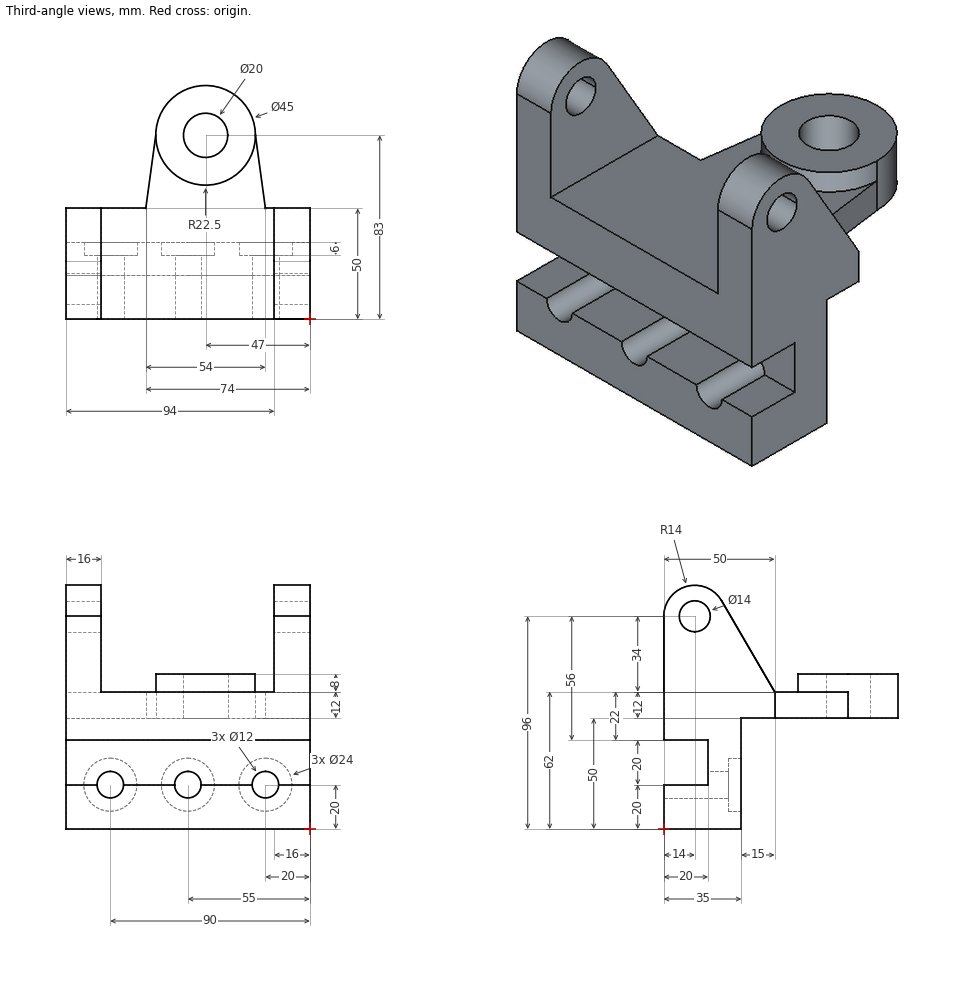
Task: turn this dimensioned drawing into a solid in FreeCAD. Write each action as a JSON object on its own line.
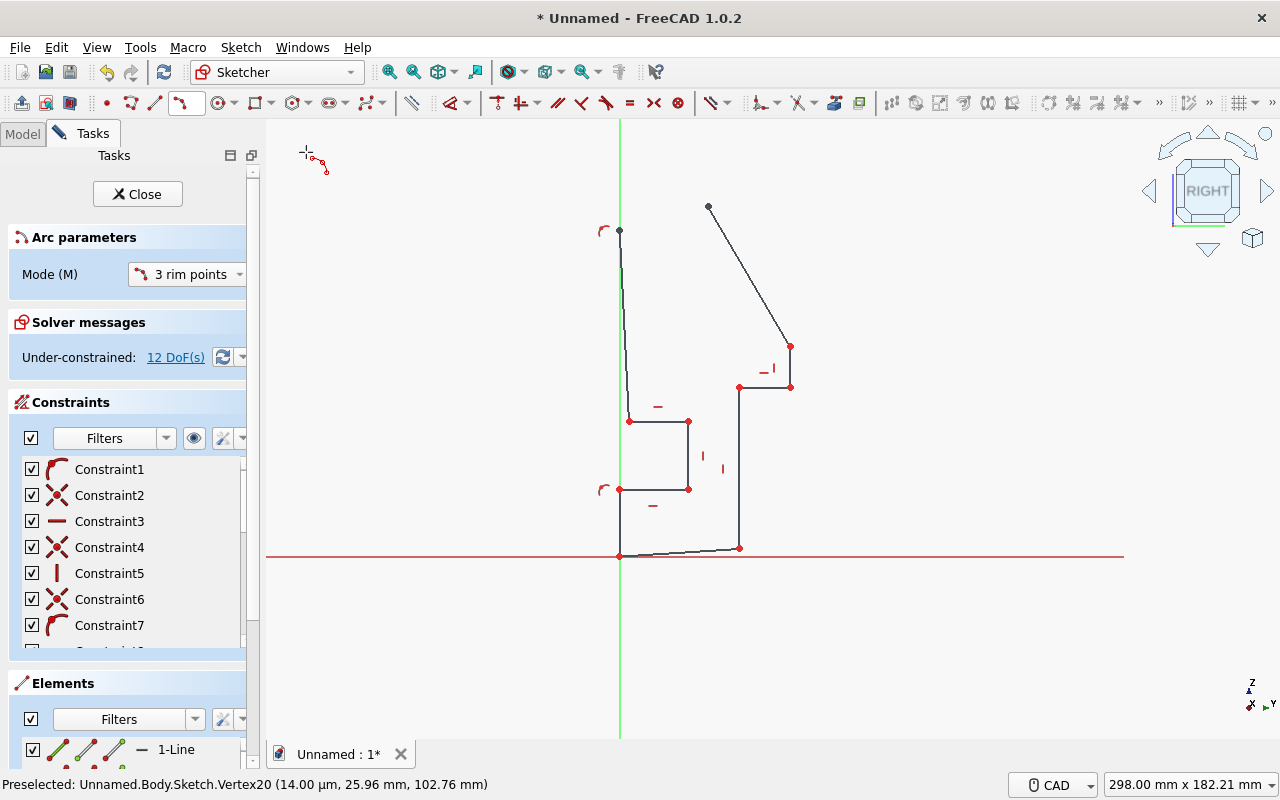
{"action": "left_click", "coordinate": [708, 207]}
{"action": "left_click", "coordinate": [620, 231]}
{"action": "left_click", "coordinate": [655, 184]}
{"action": "key", "text": "Escape"}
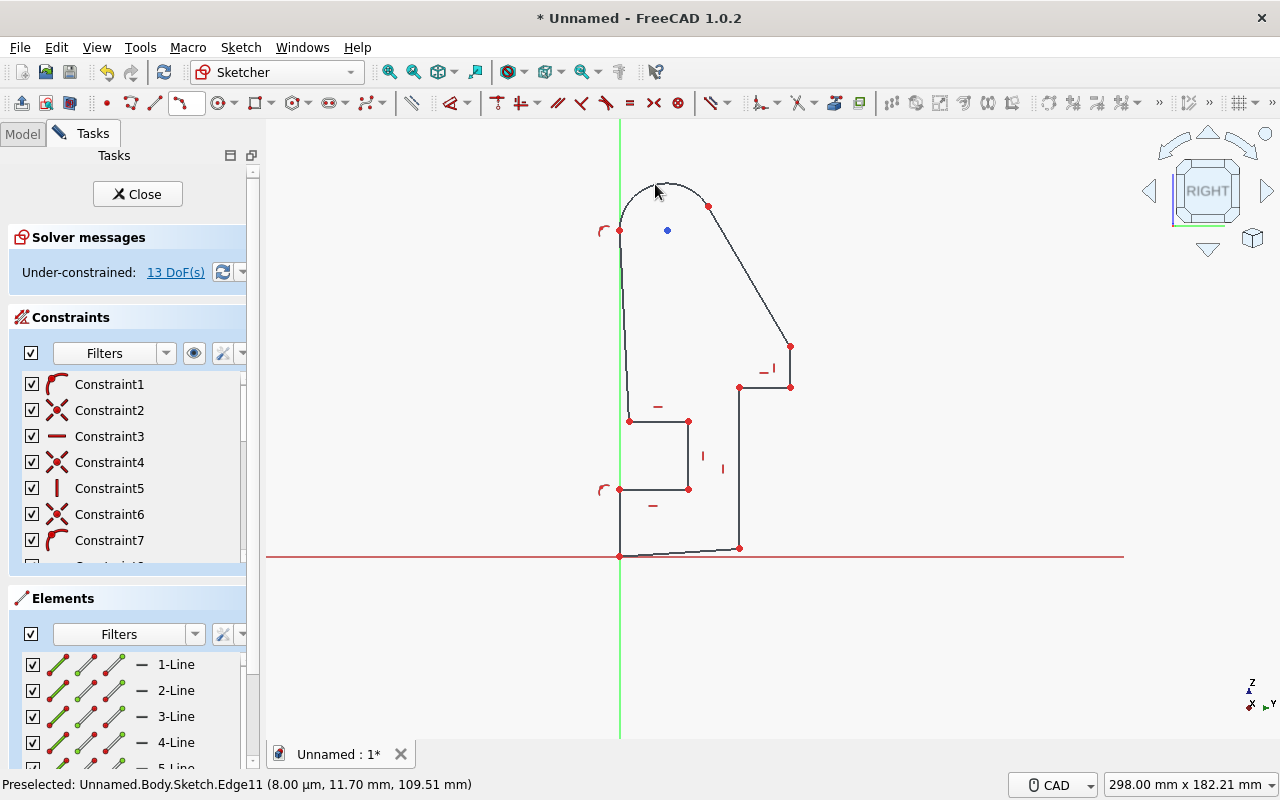
{"action": "left_click", "coordinate": [622, 288]}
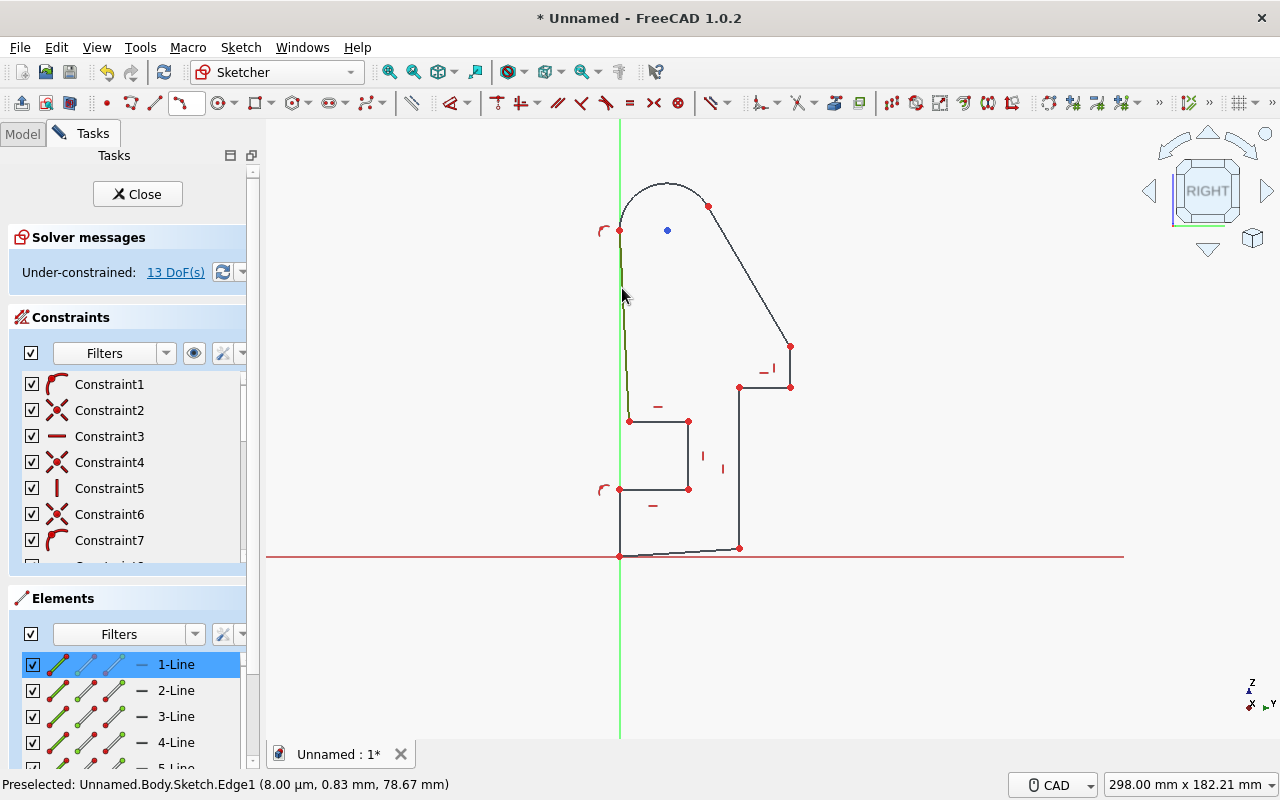
{"action": "left_click", "coordinate": [679, 185]}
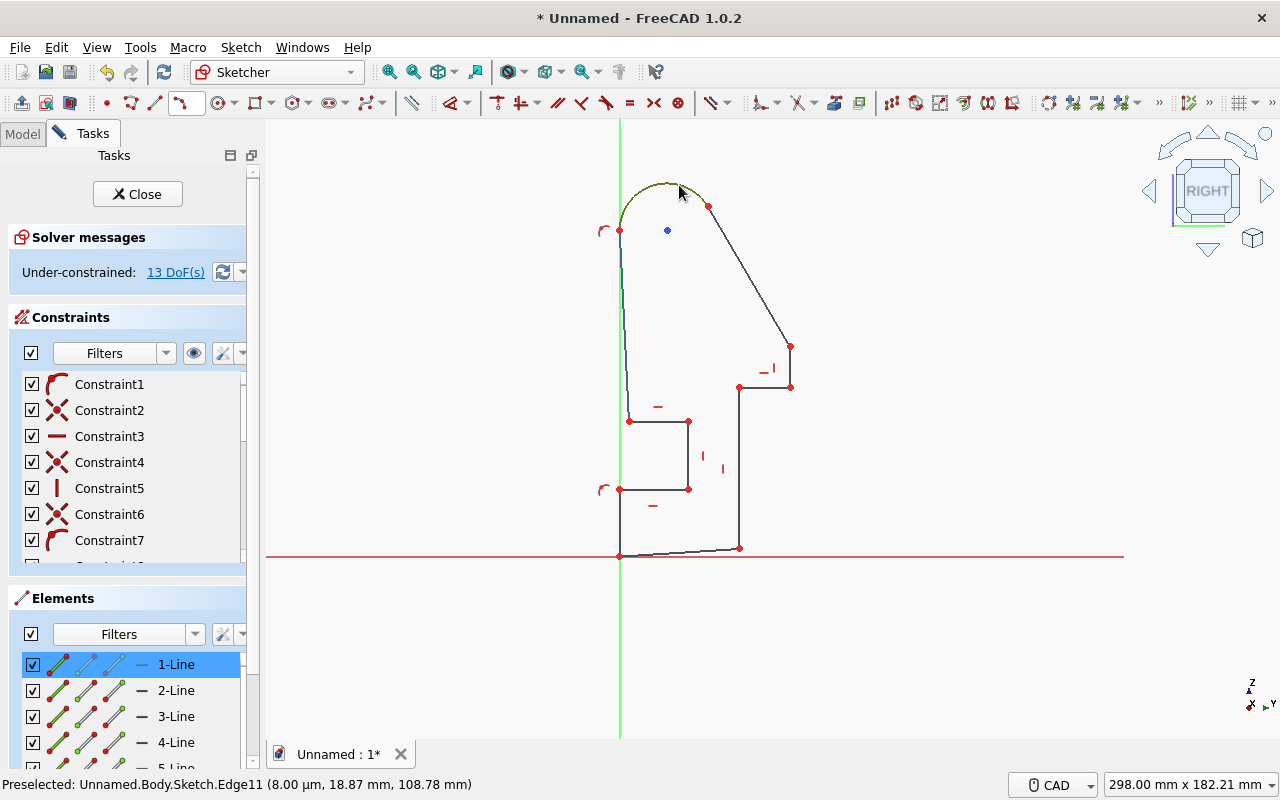
{"action": "left_click", "coordinate": [606, 104]}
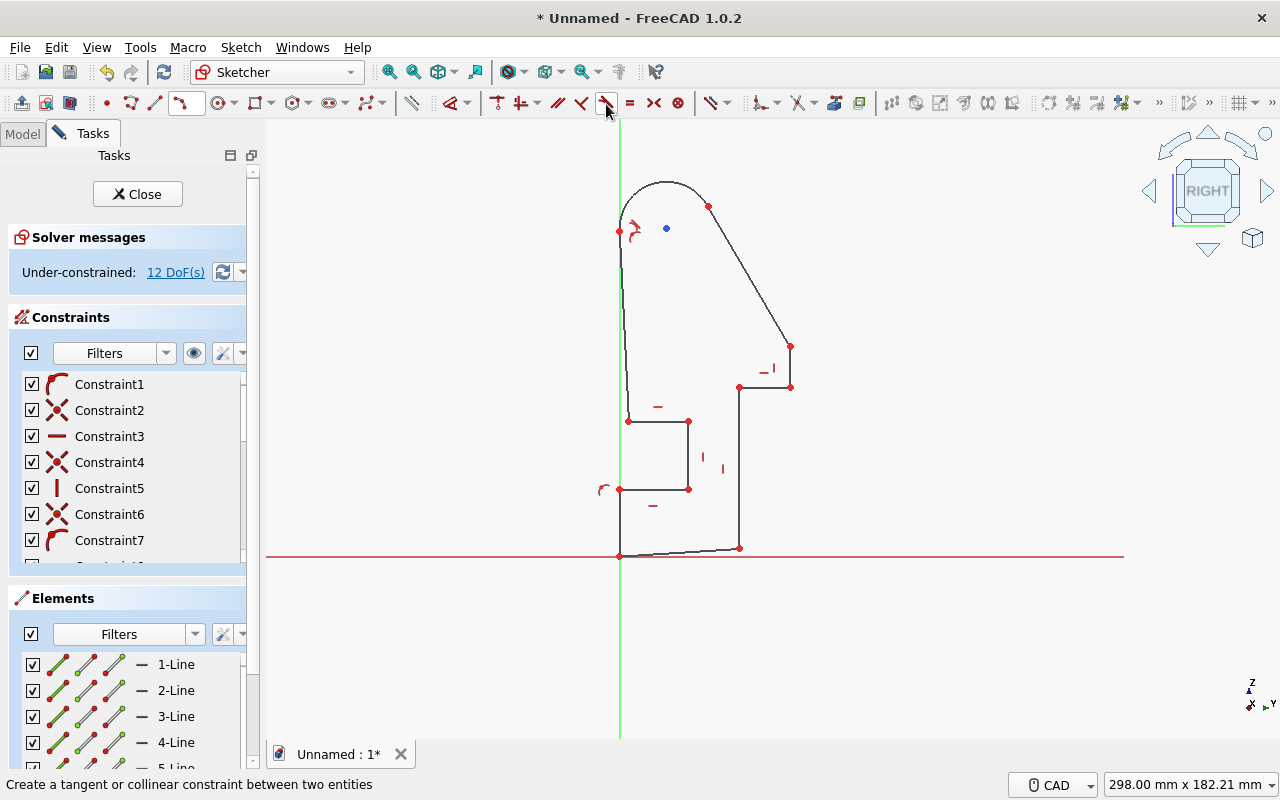
{"action": "left_click", "coordinate": [765, 305]}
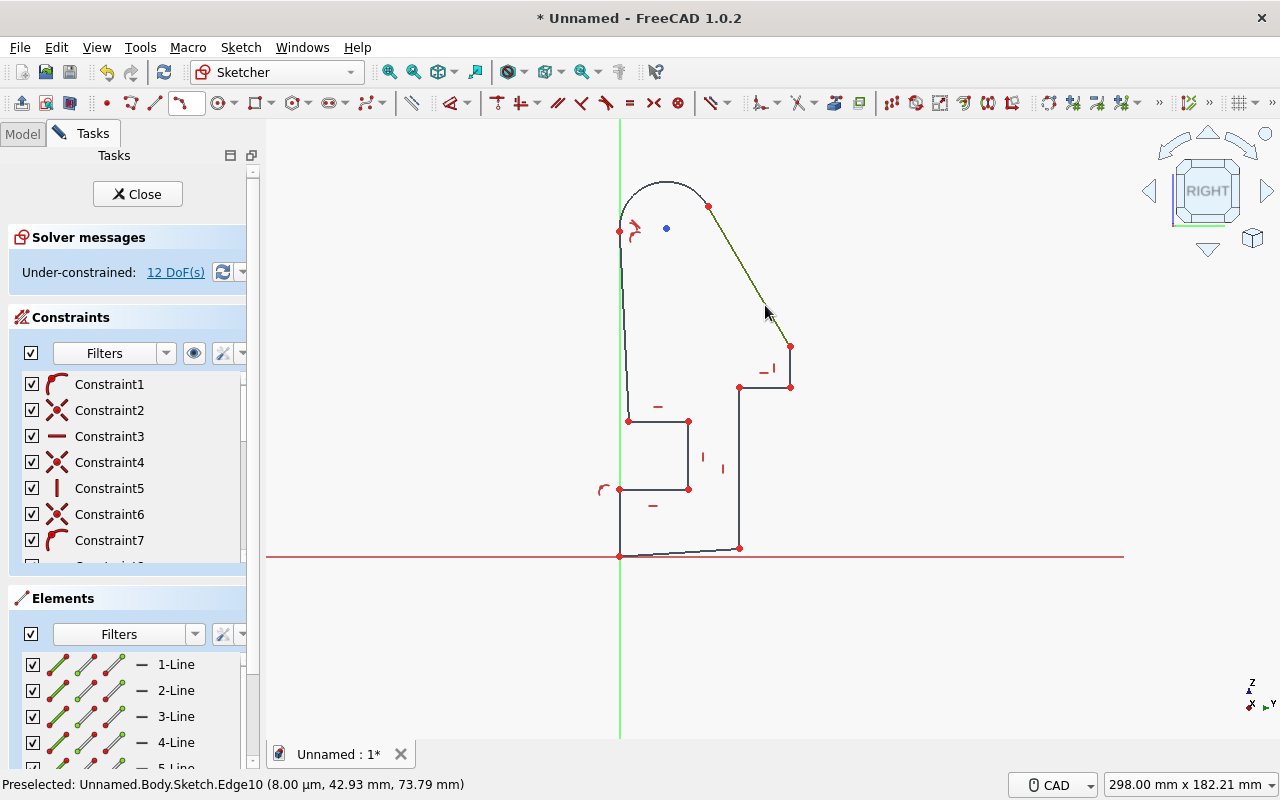
{"action": "left_click", "coordinate": [679, 184]}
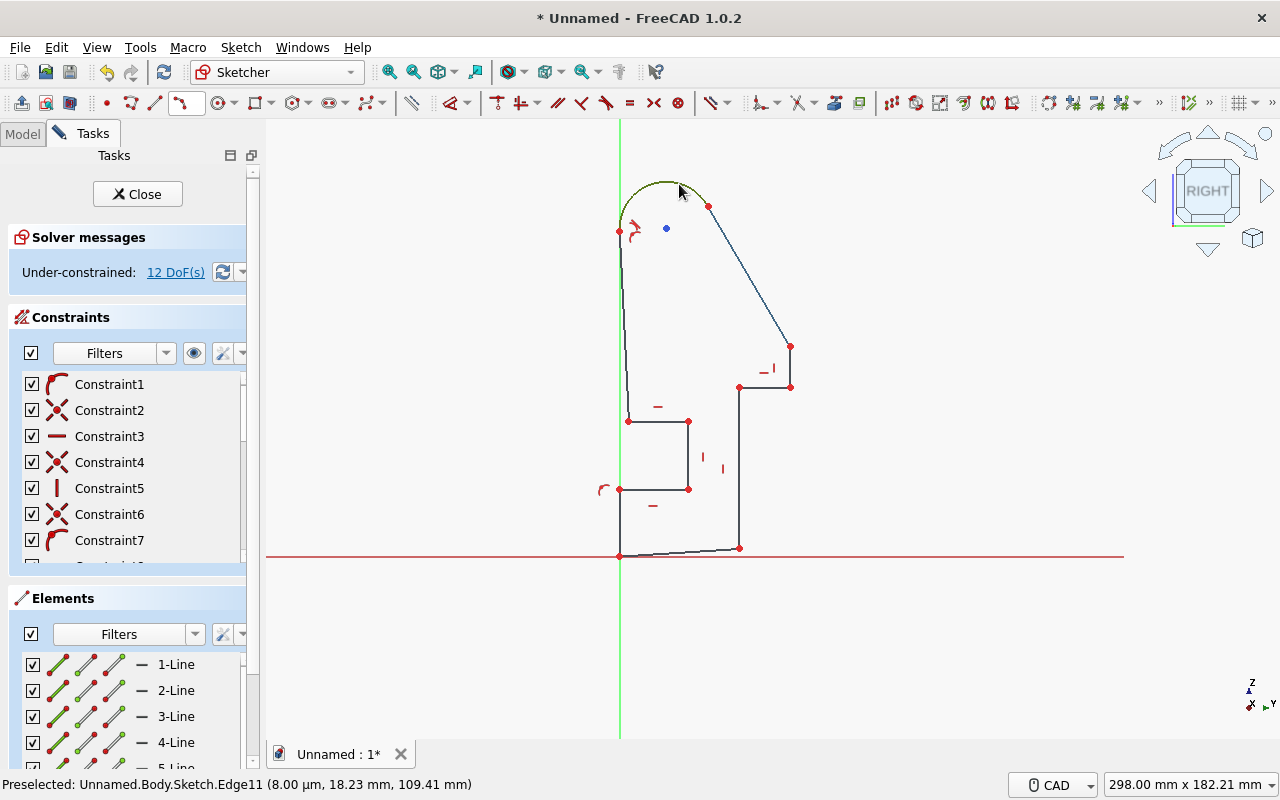
{"action": "left_click", "coordinate": [606, 104]}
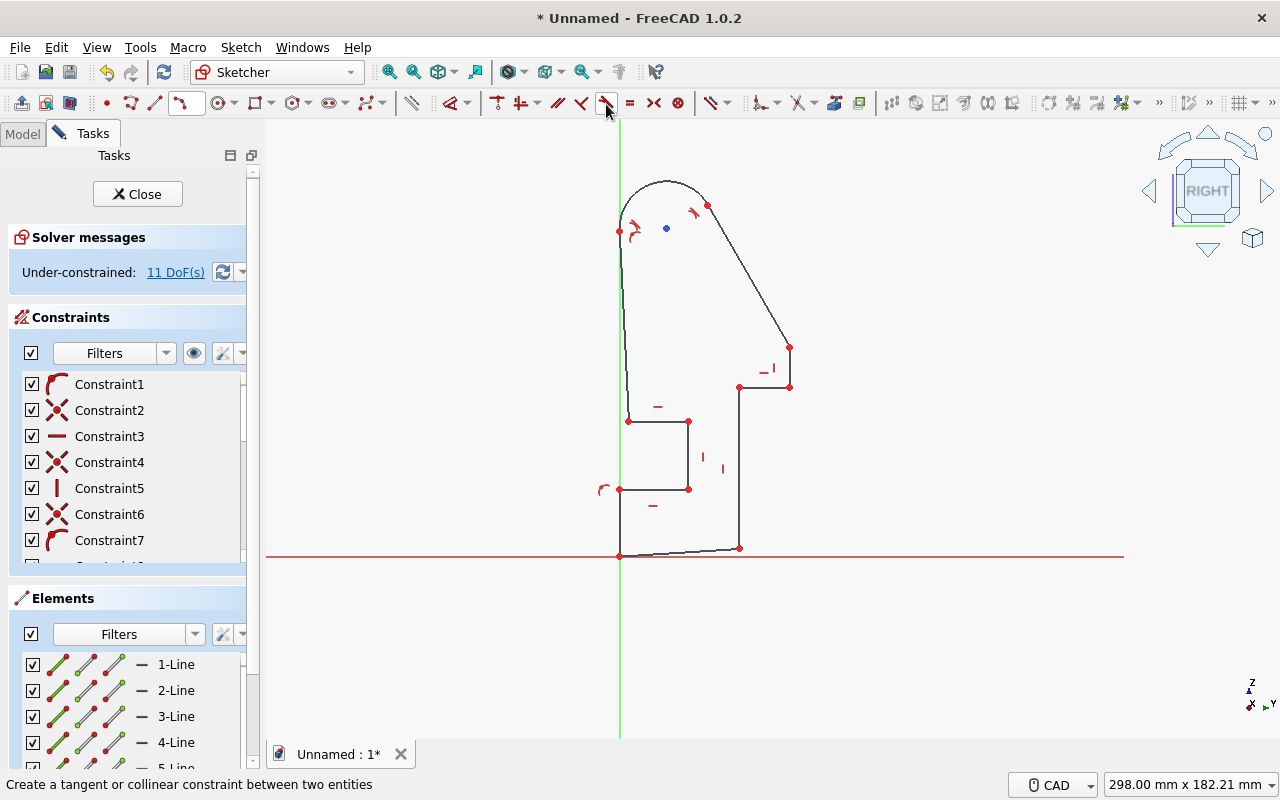
{"action": "left_click", "coordinate": [622, 288]}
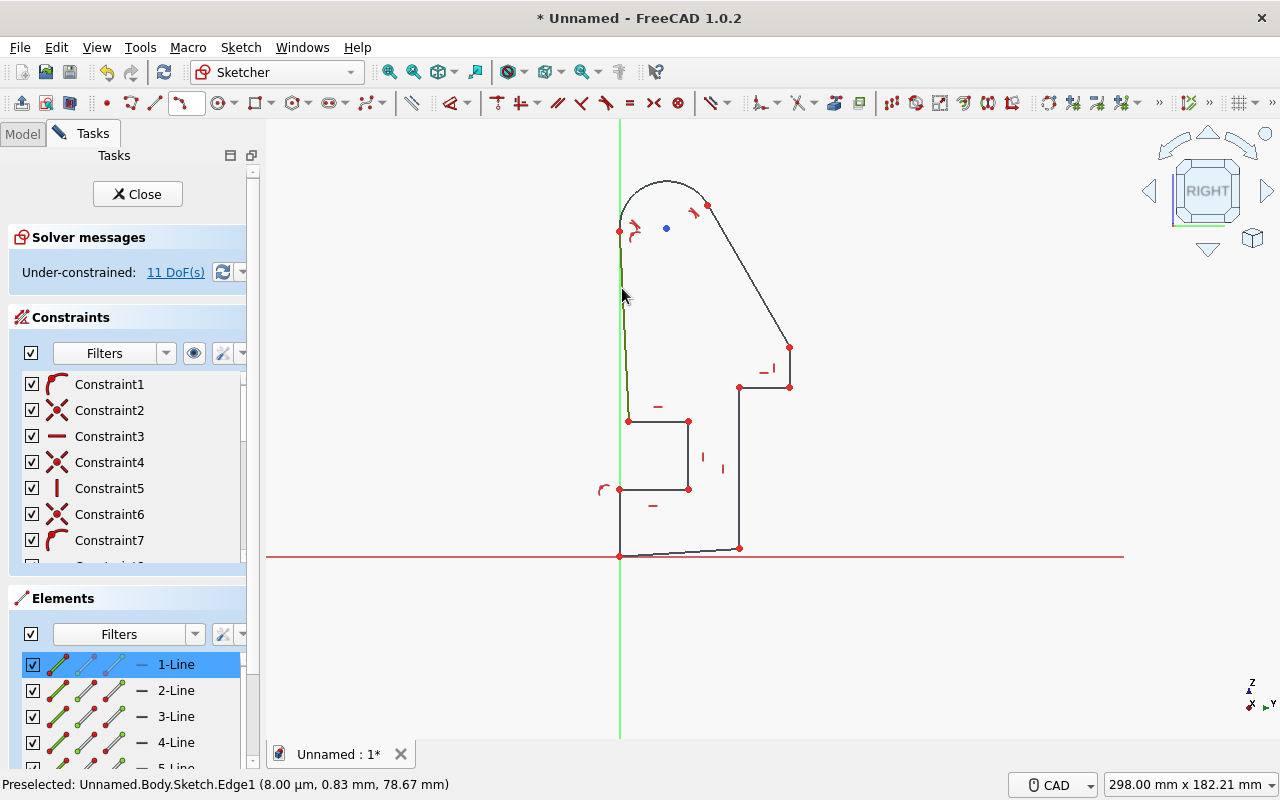
{"action": "key", "text": "v"}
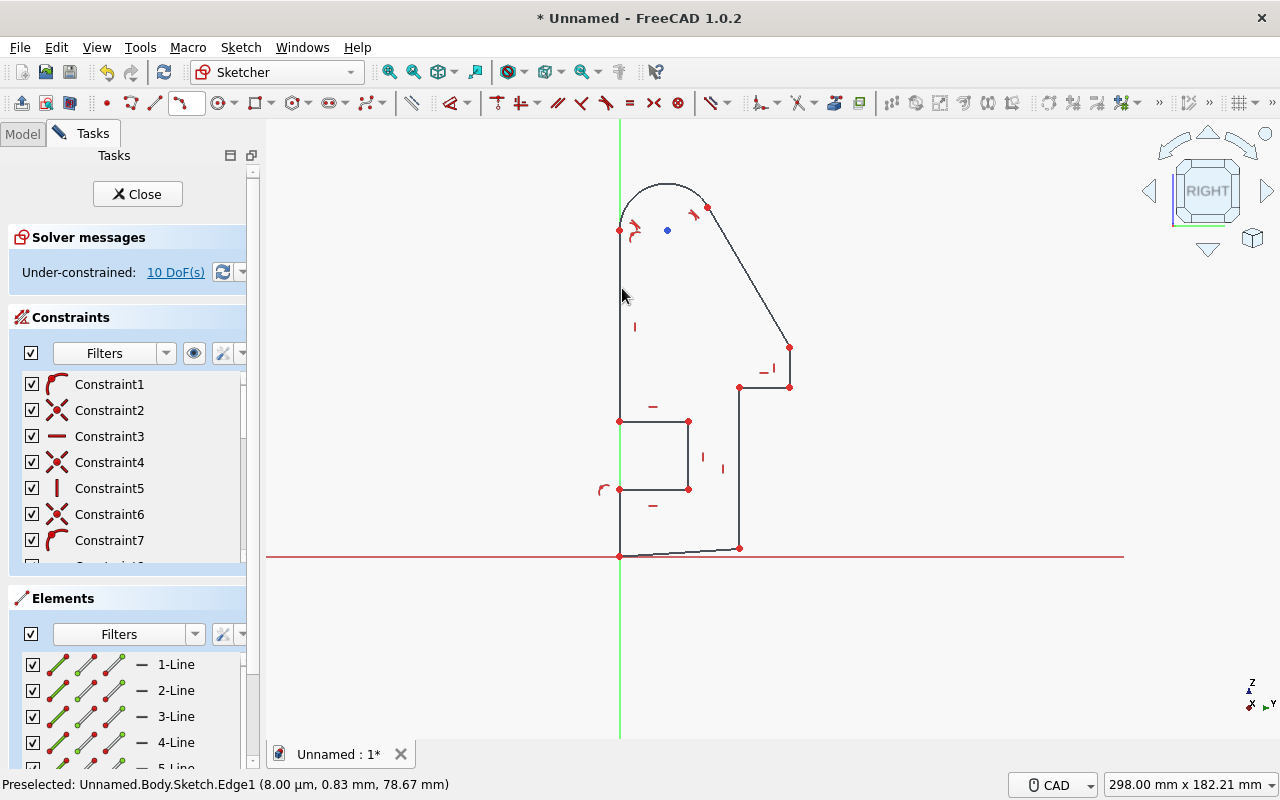
{"action": "left_click", "coordinate": [655, 554]}